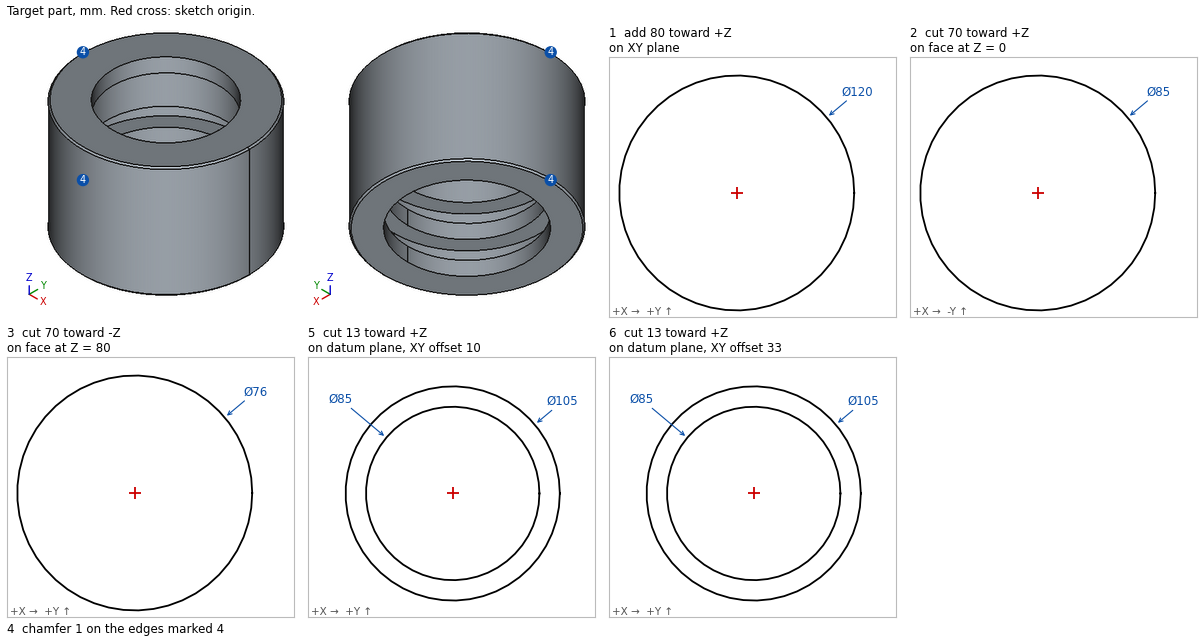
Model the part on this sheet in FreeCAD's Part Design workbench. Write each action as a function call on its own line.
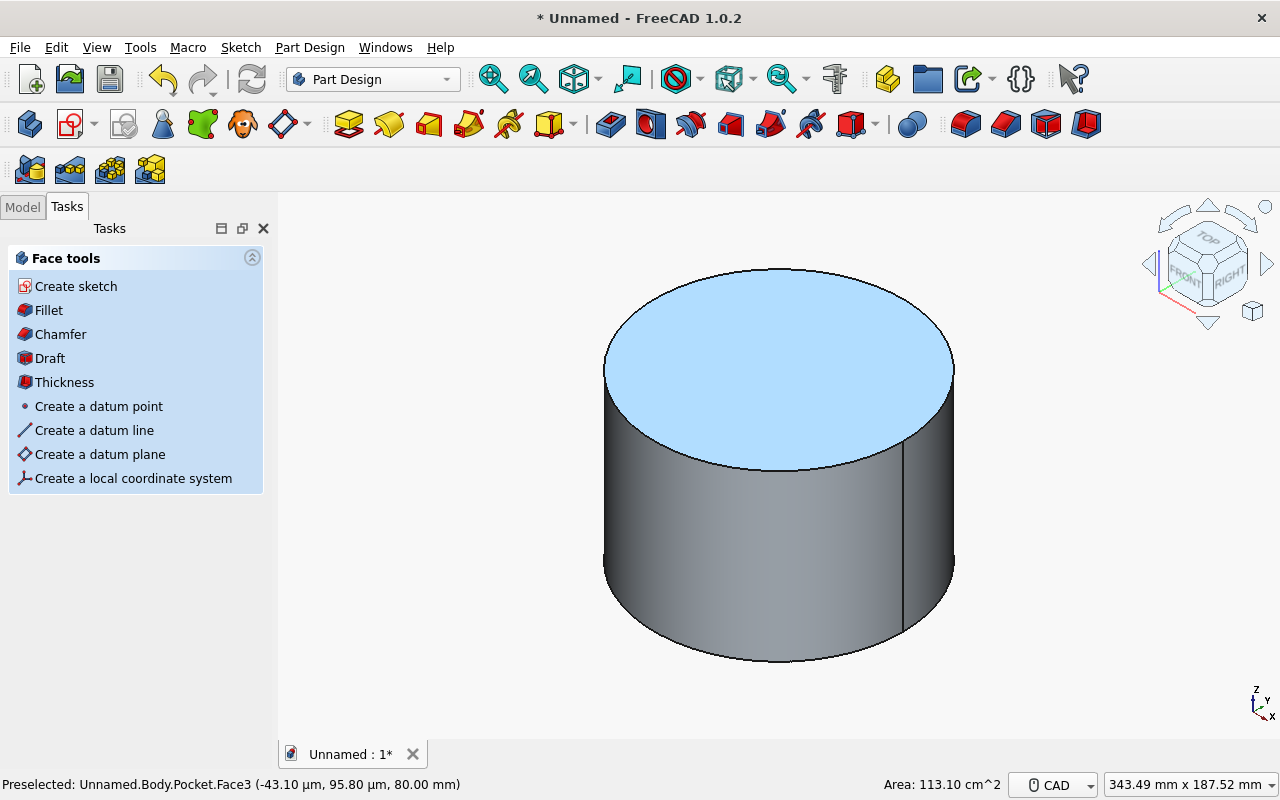
click(70, 124)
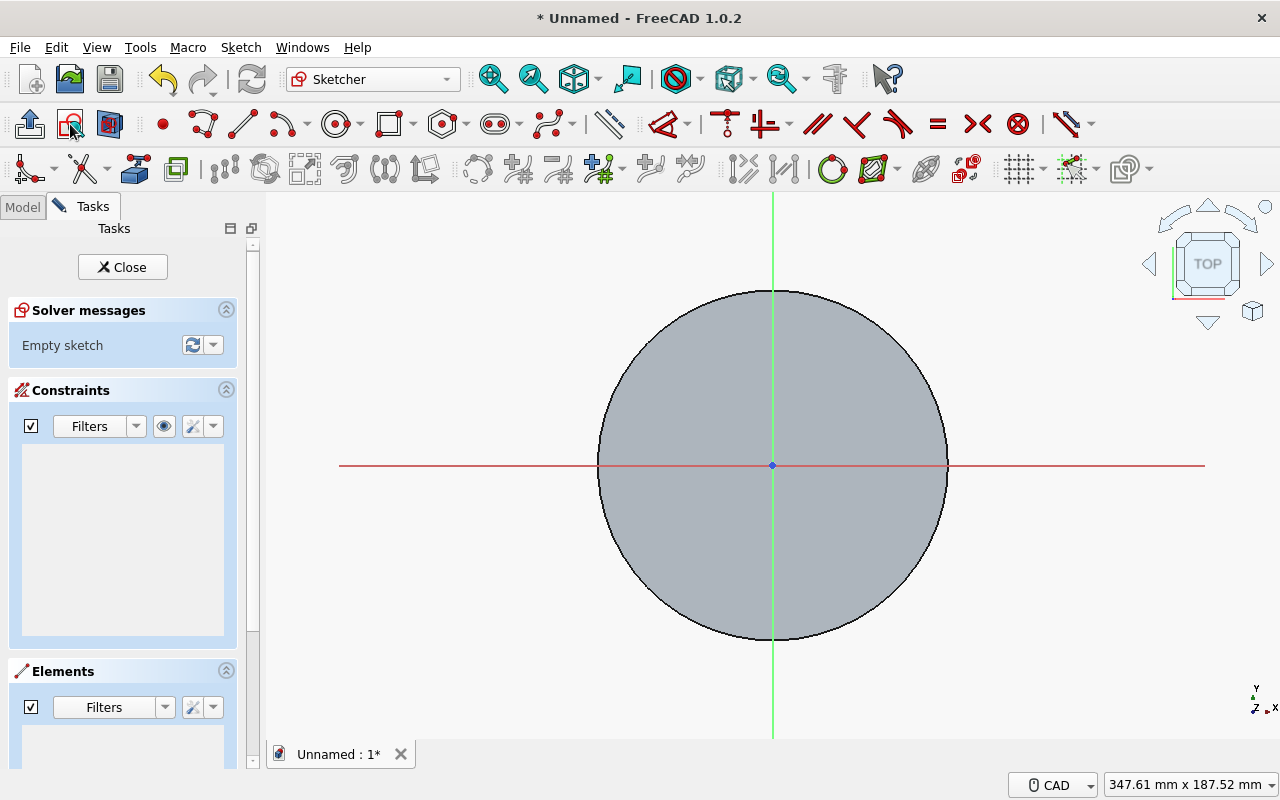
scroll(912, 465, up, 2)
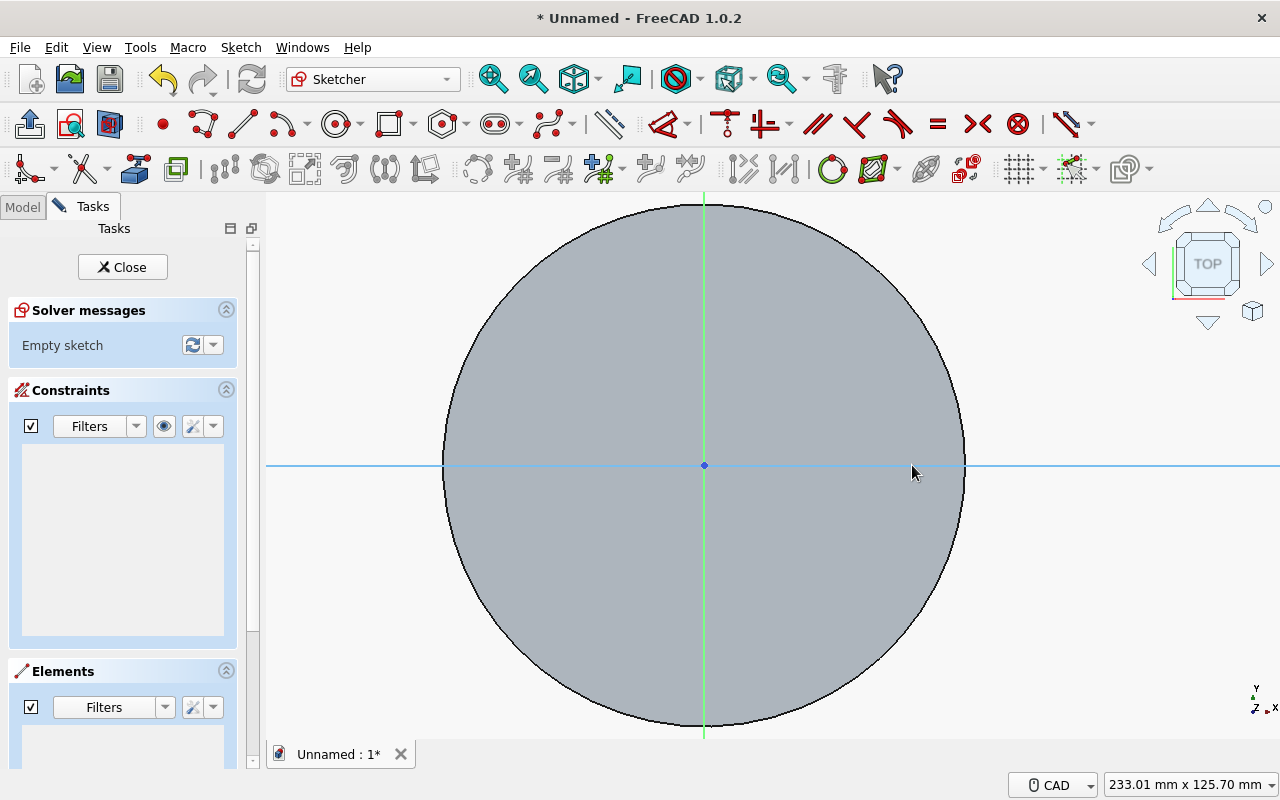
click(336, 124)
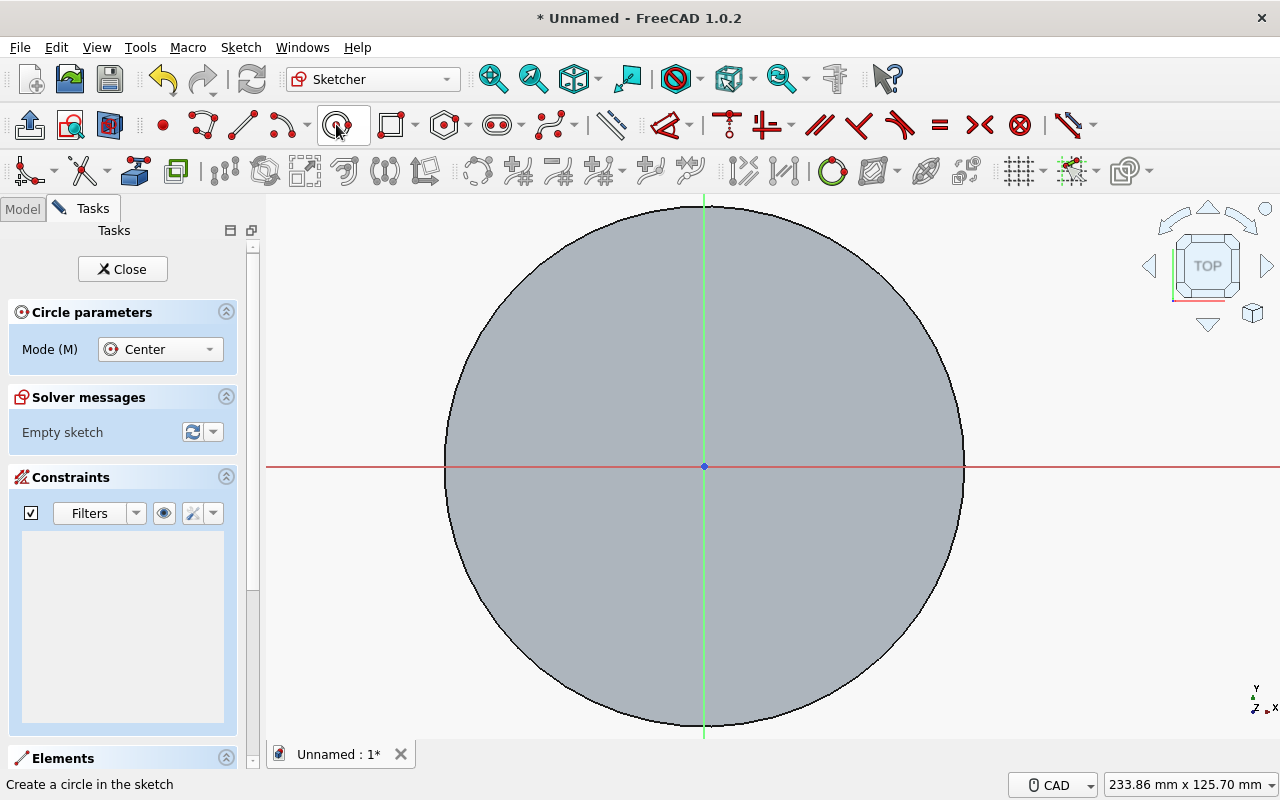
click(704, 466)
click(821, 350)
key(Escape)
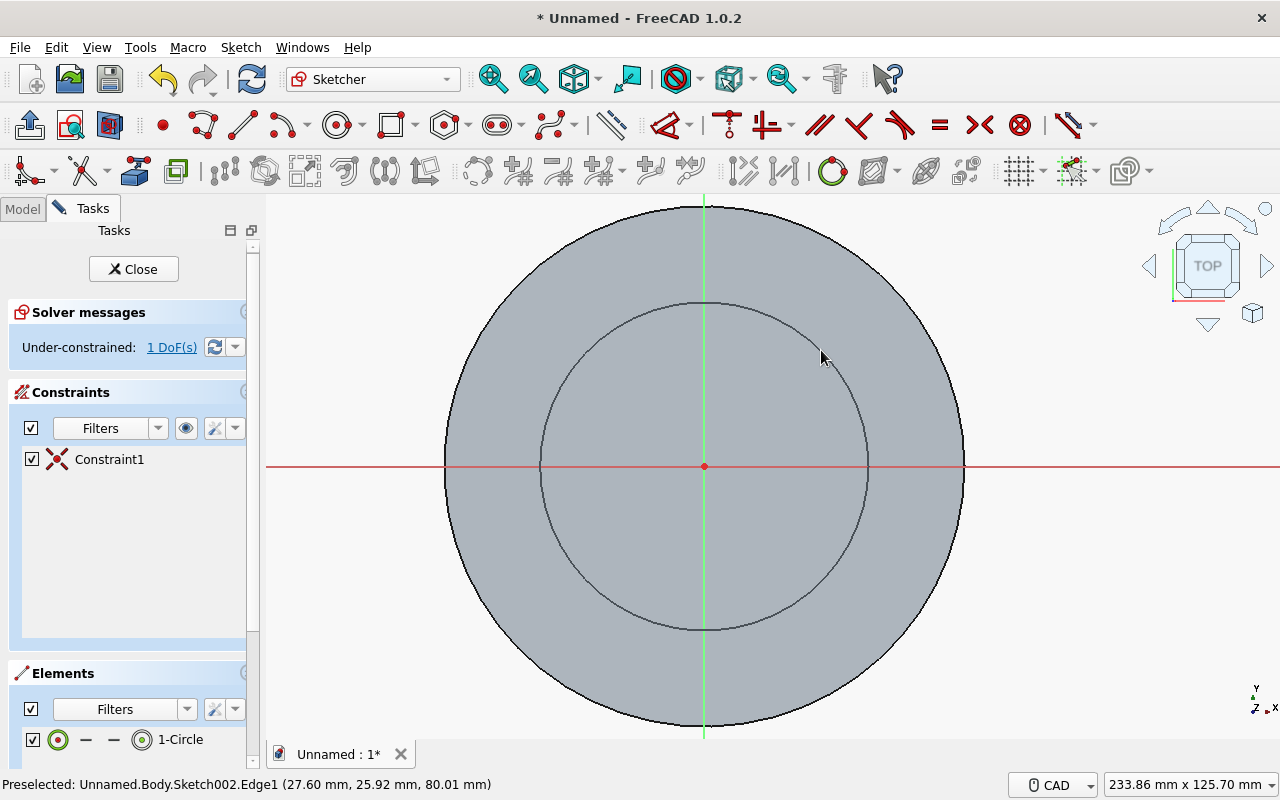
click(820, 350)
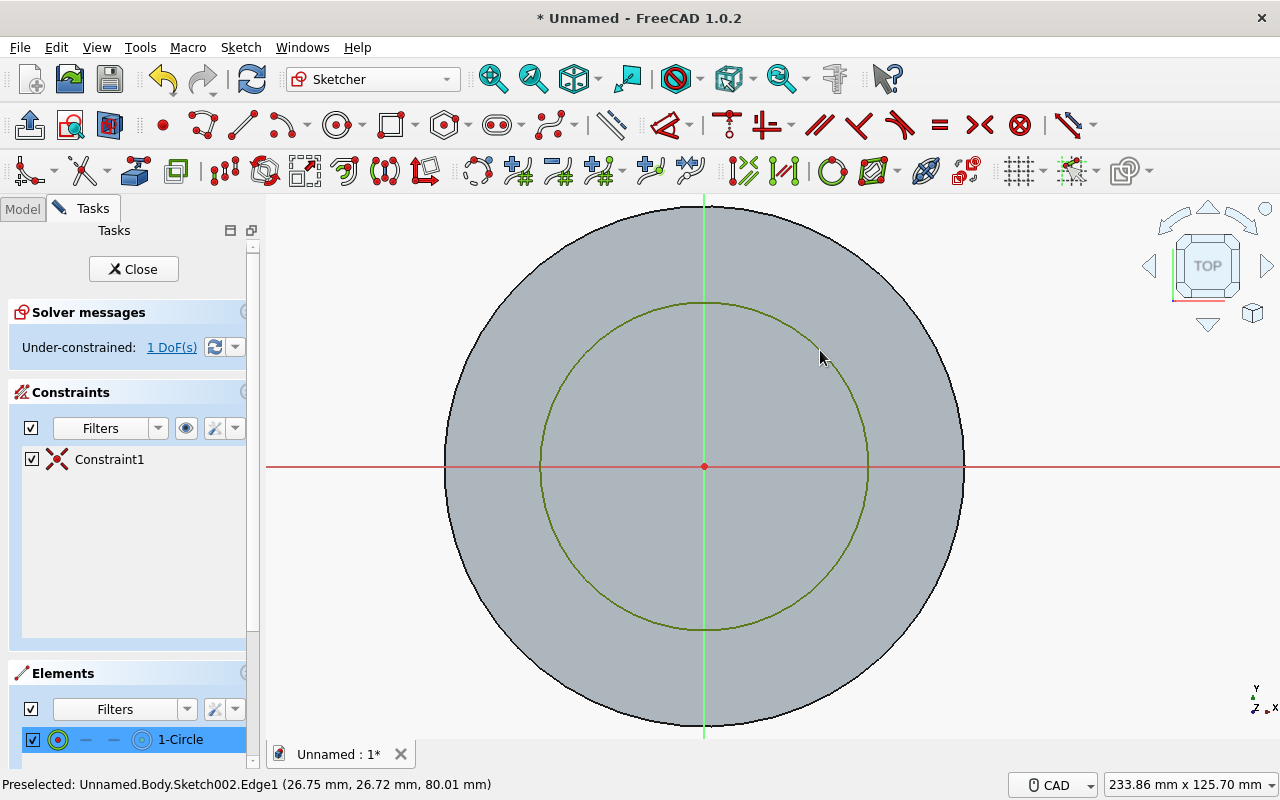
click(692, 126)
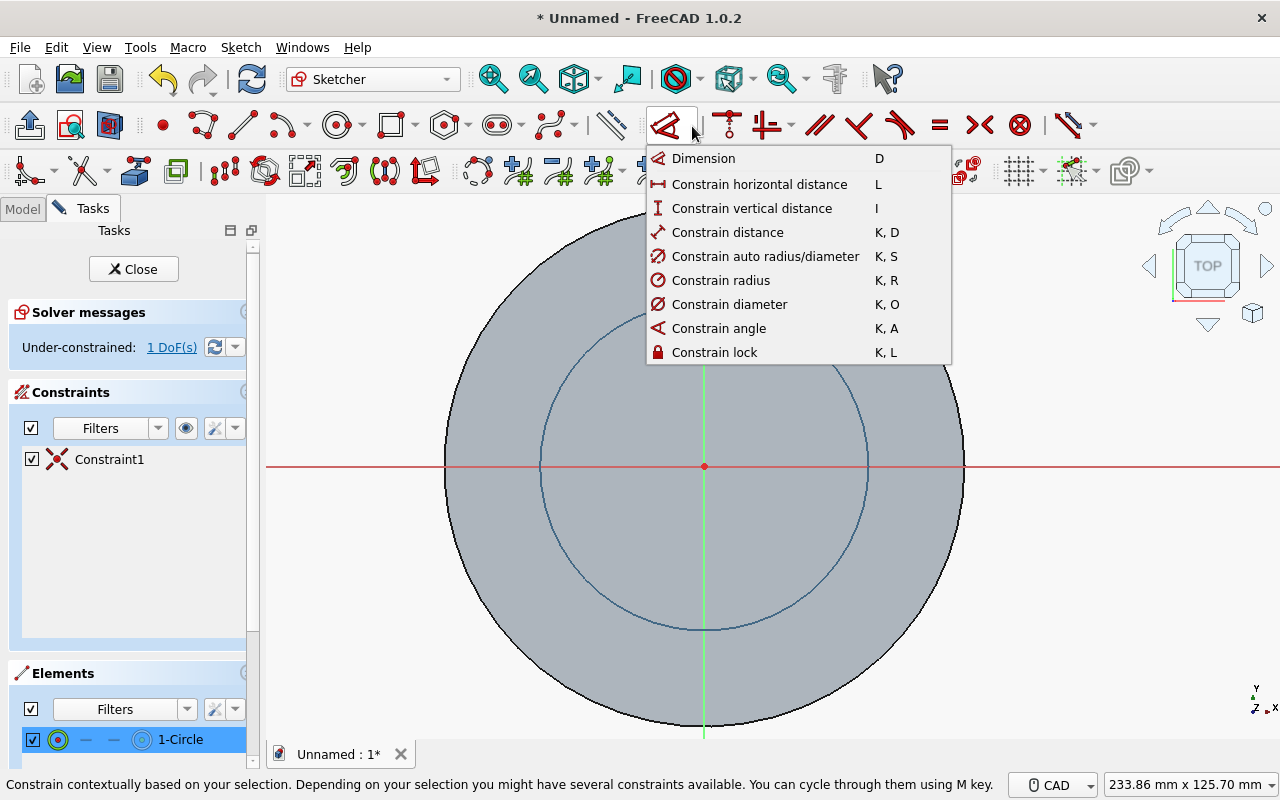
click(799, 304)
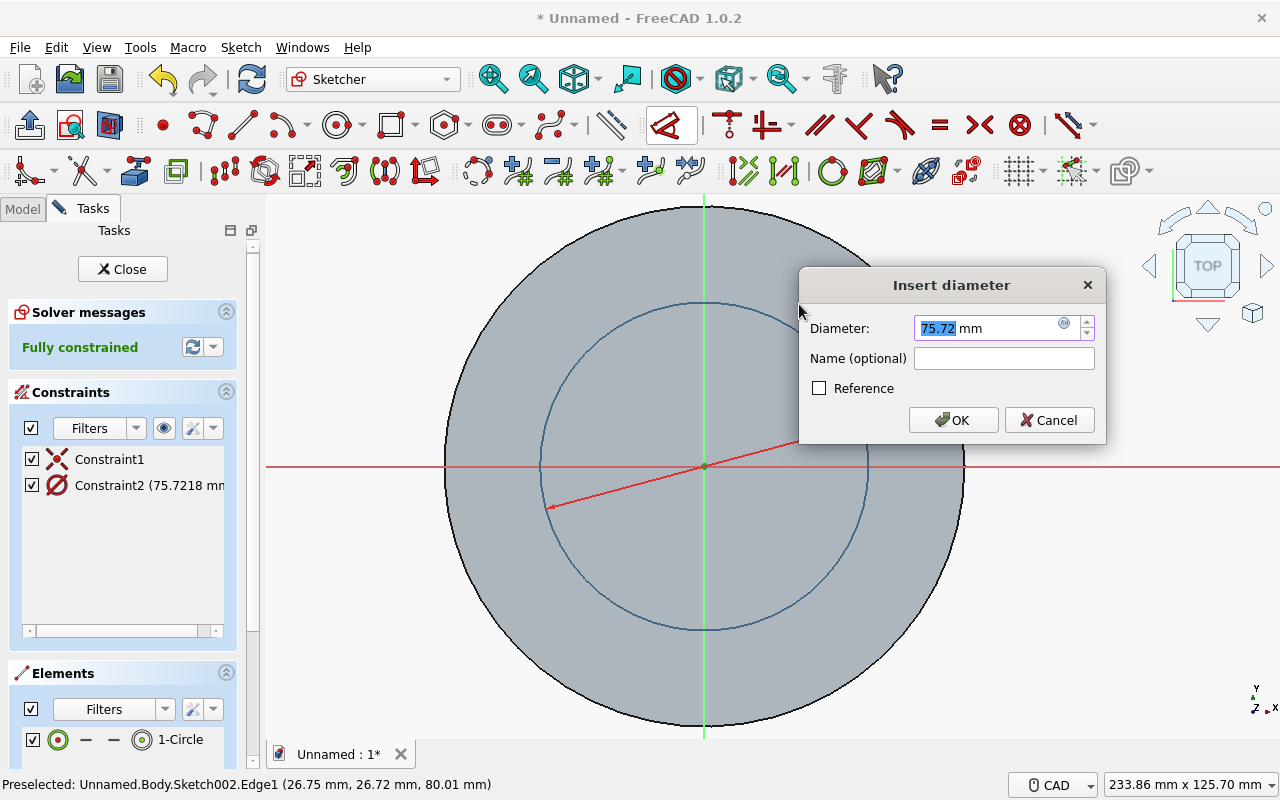
text(76)
key(Return)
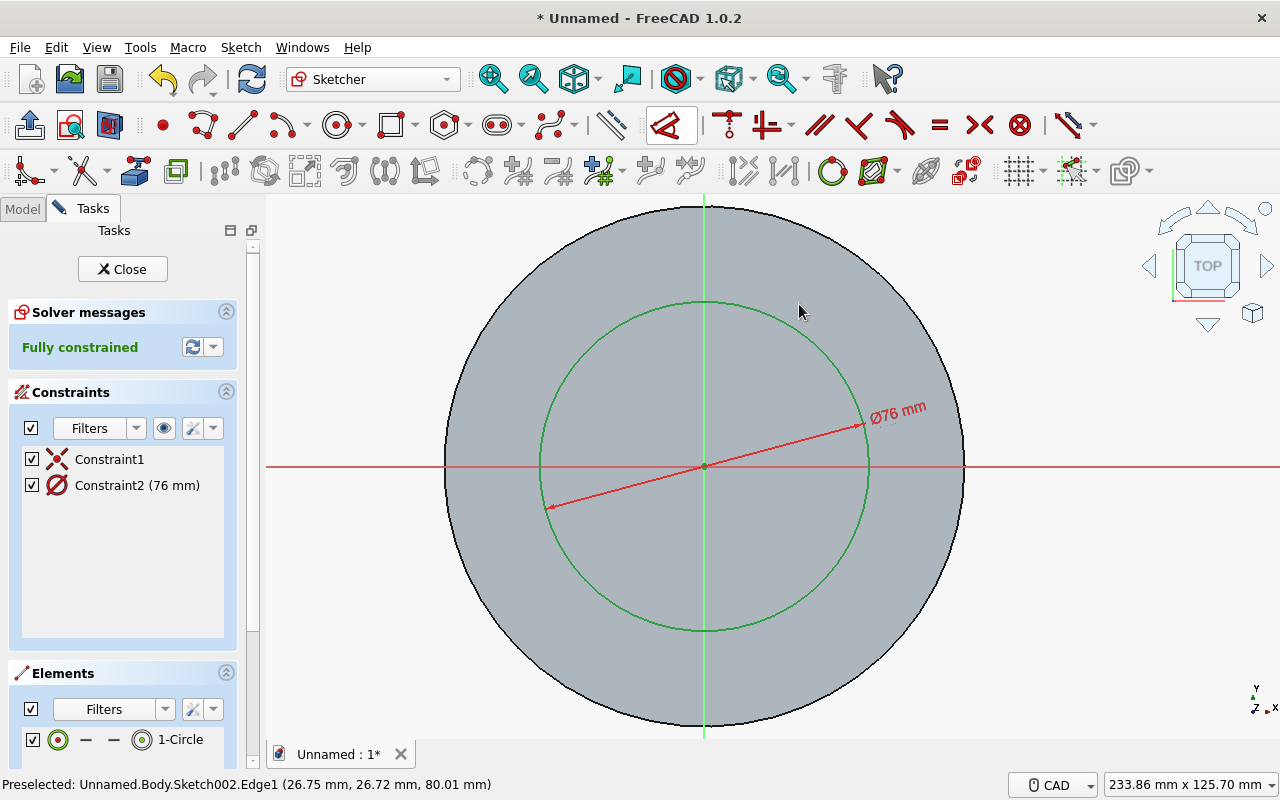
click(123, 269)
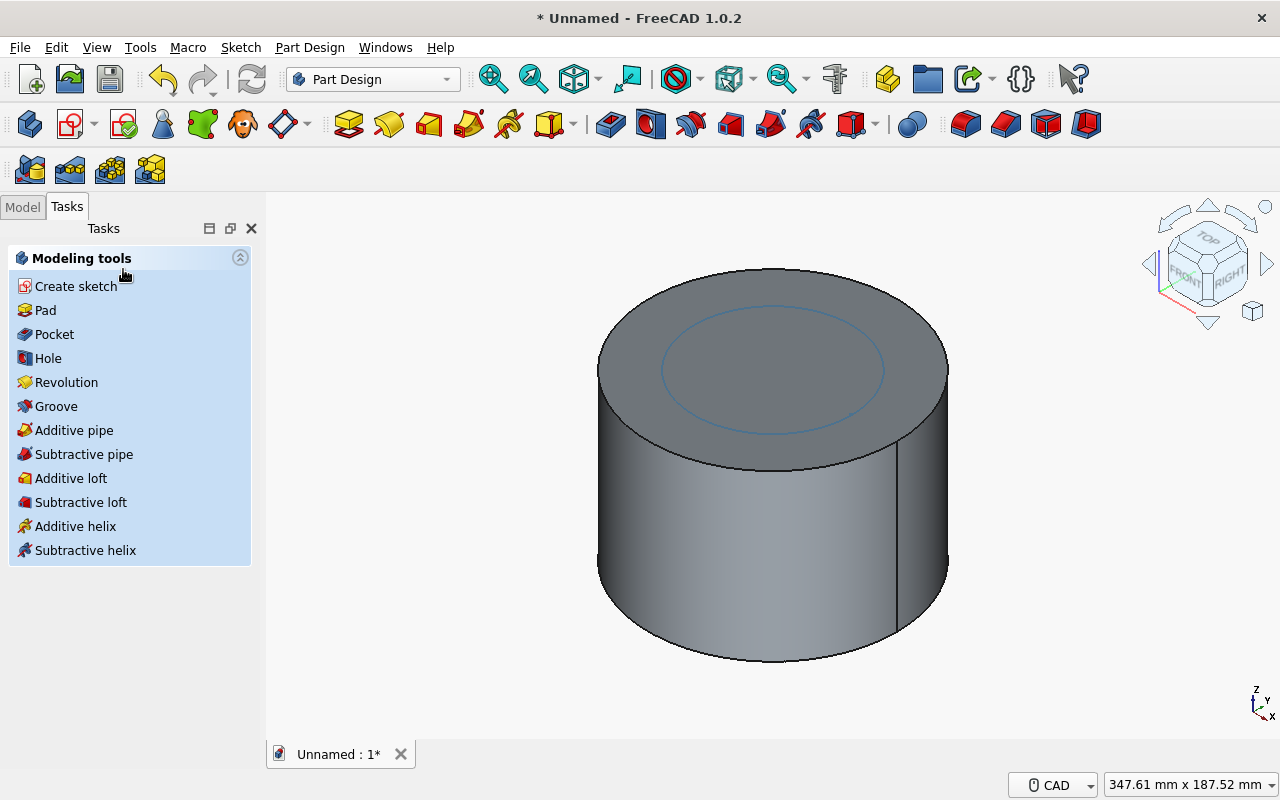
click(612, 124)